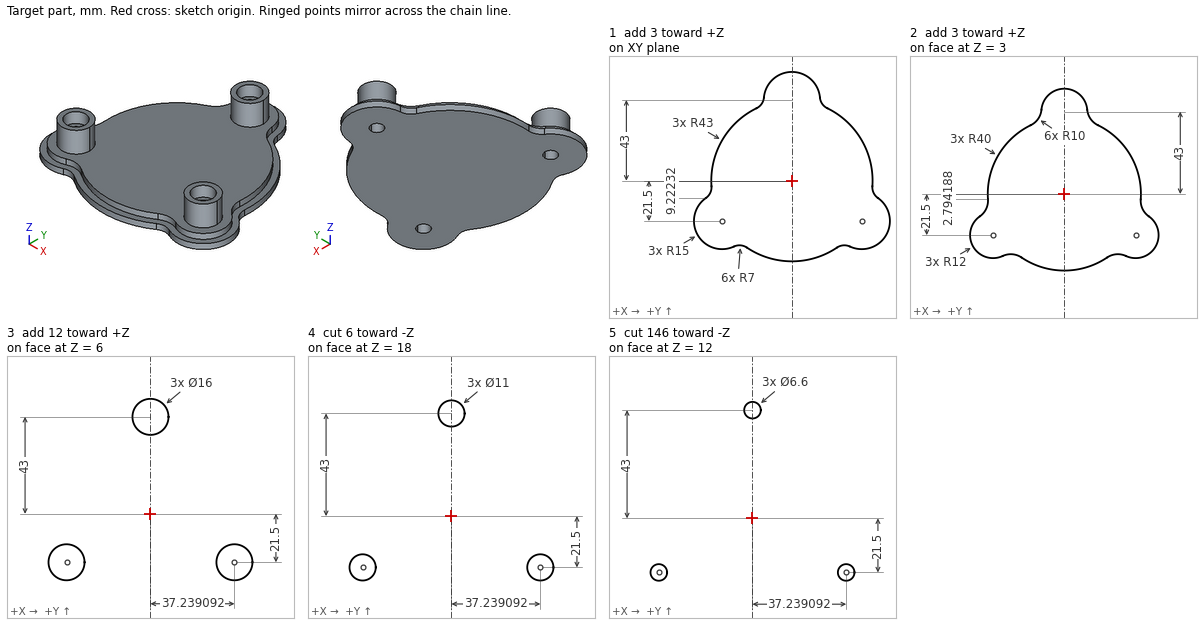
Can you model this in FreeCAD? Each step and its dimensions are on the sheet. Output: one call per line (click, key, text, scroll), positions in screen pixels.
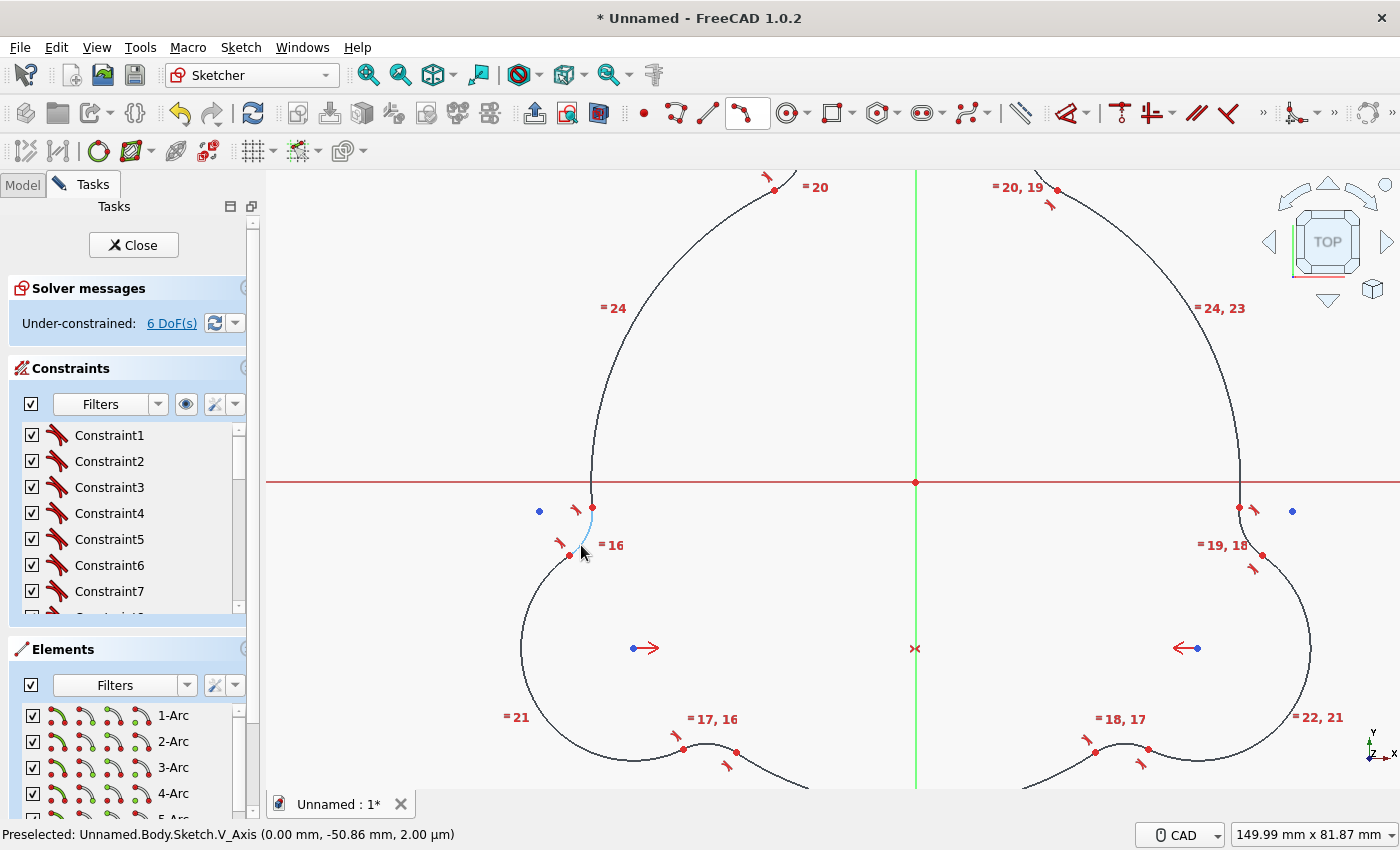
click(582, 544)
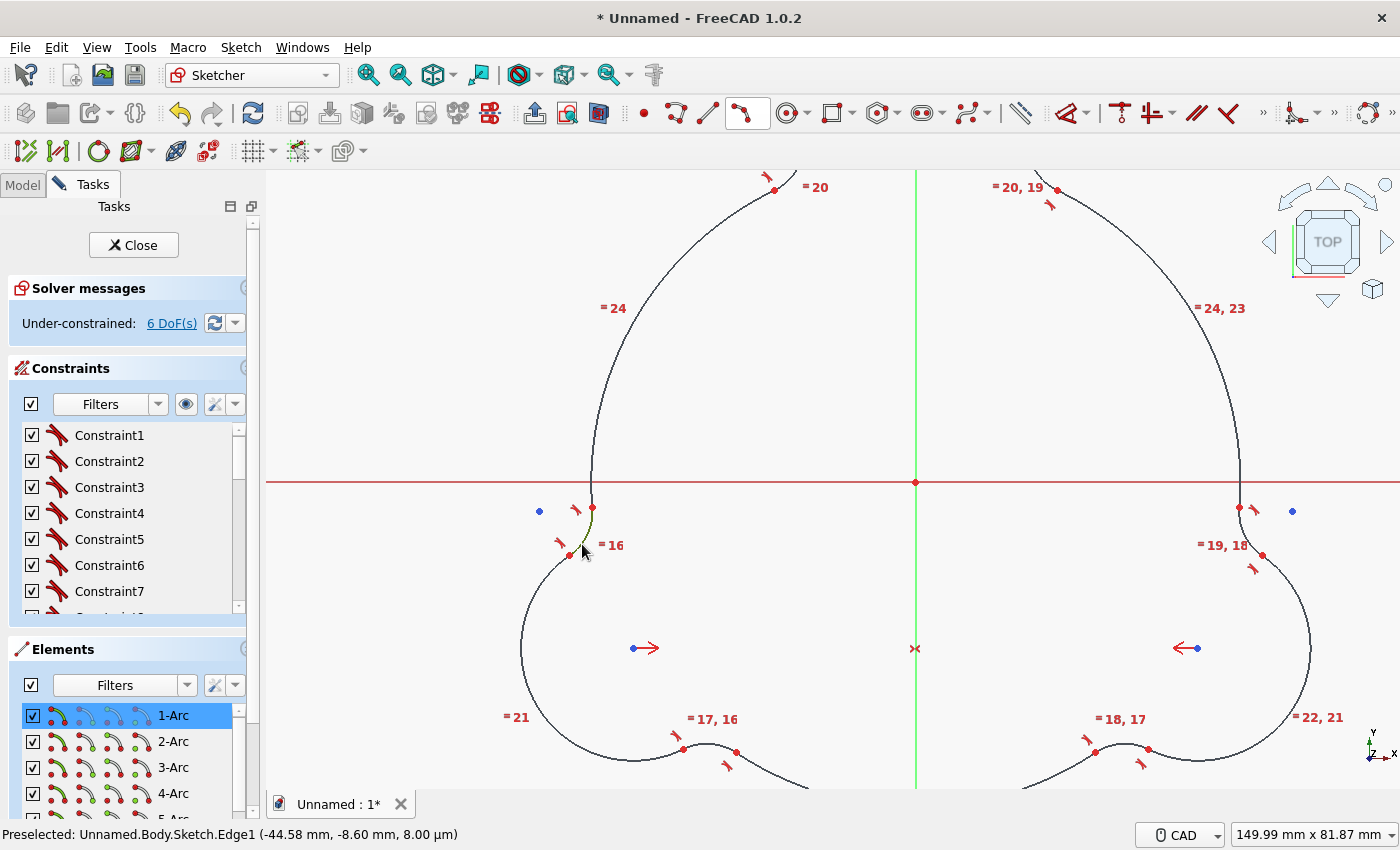
key(k)
key(r)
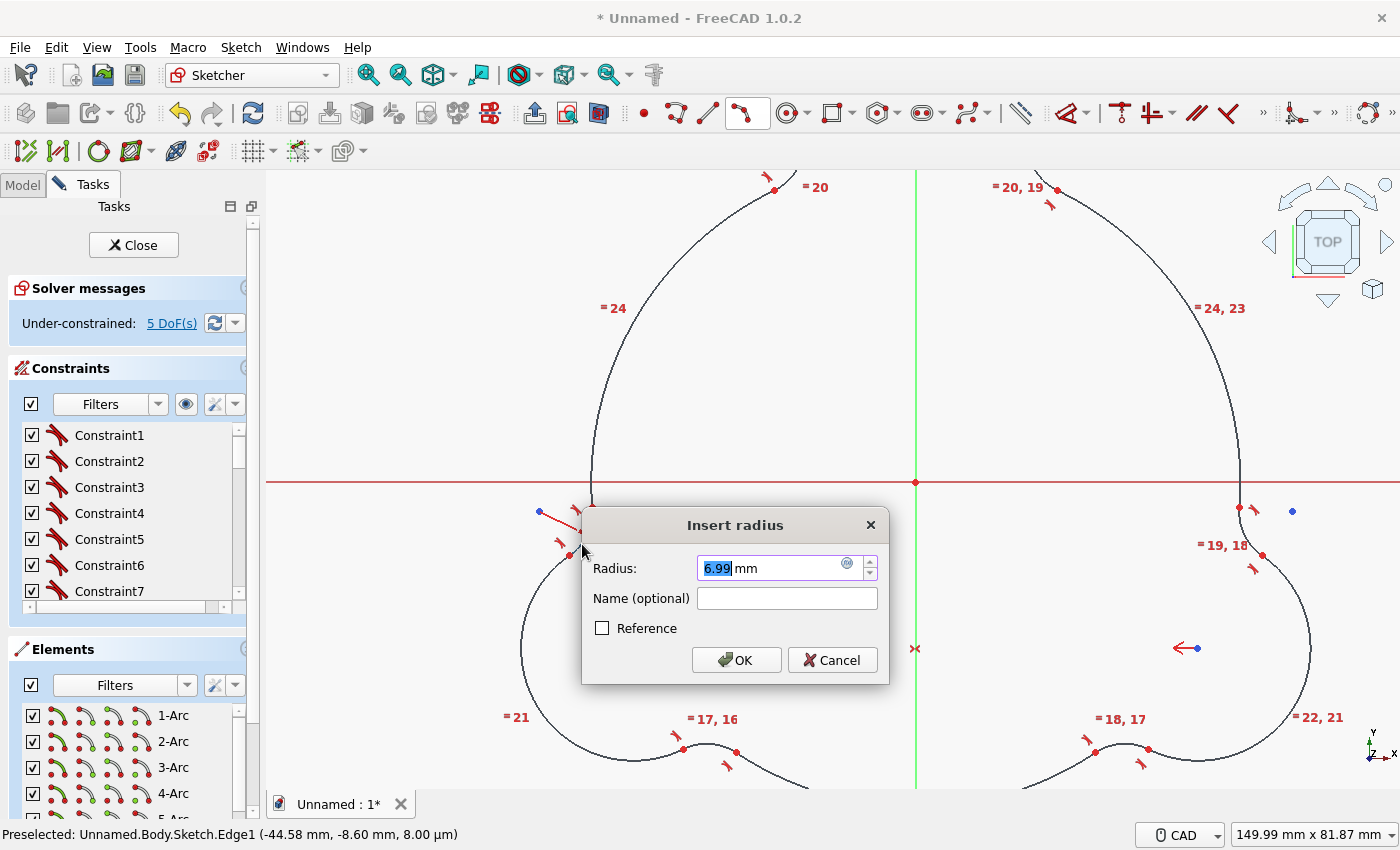
text(7)
key(Return)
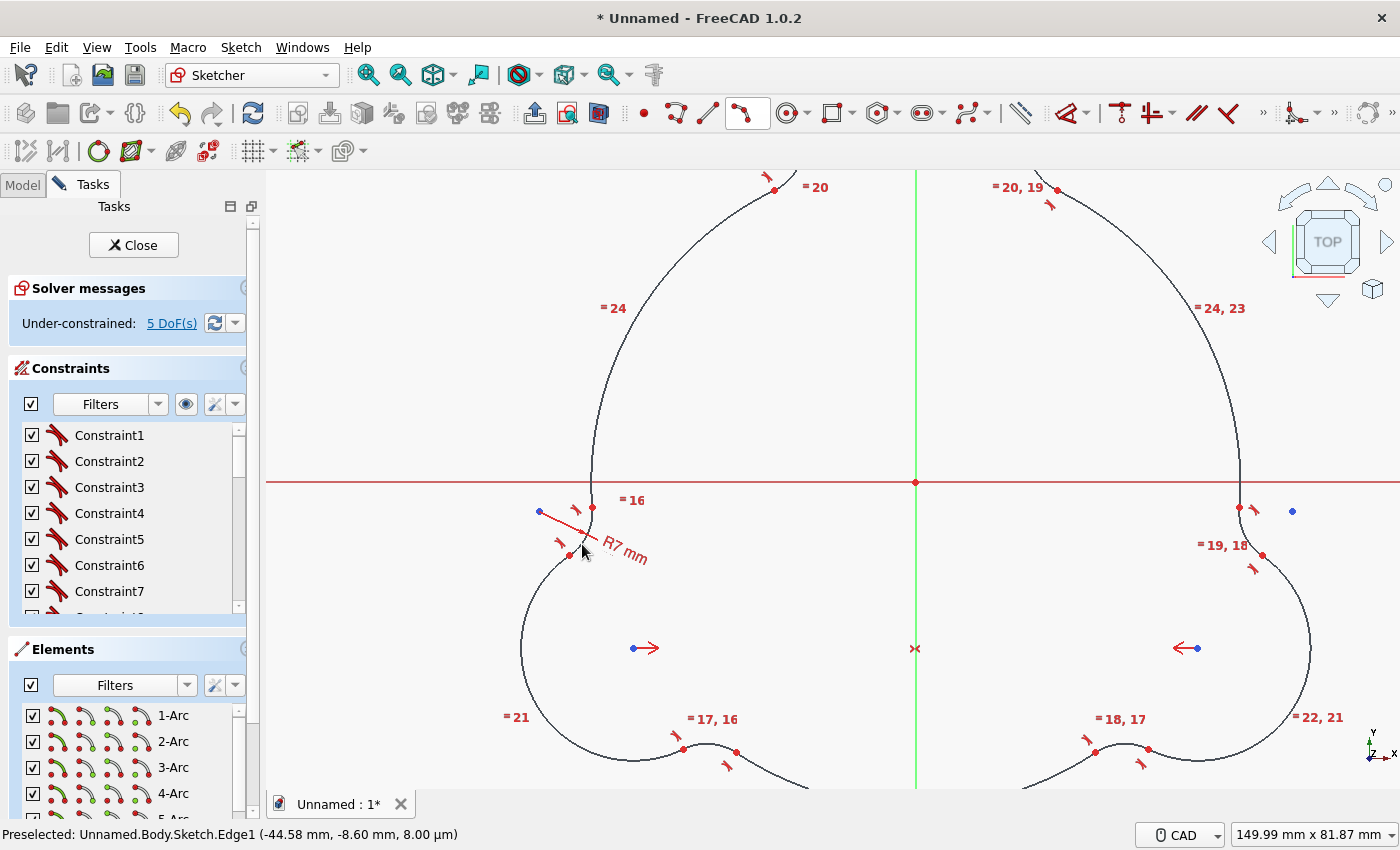
click(521, 640)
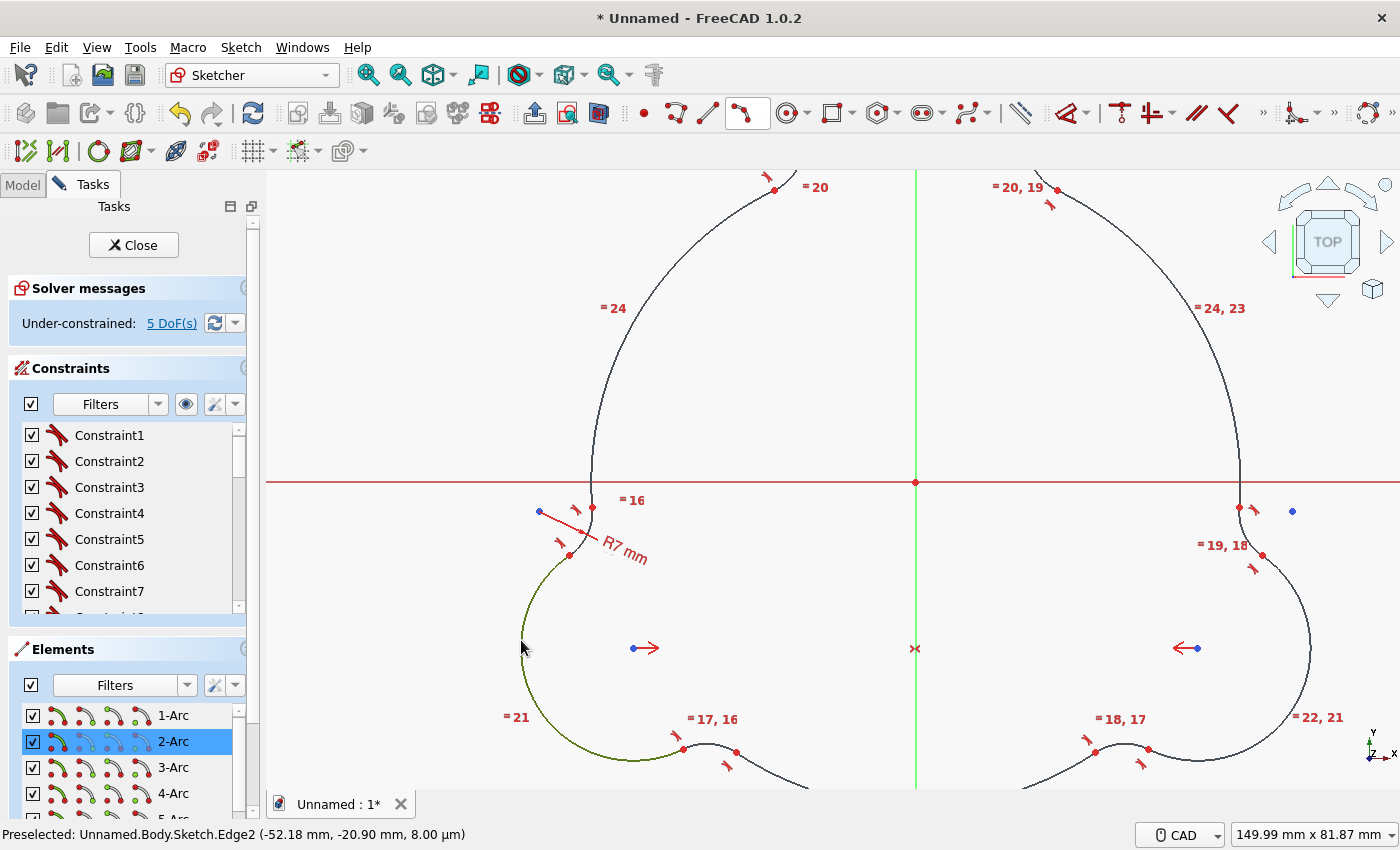
key(k)
key(r)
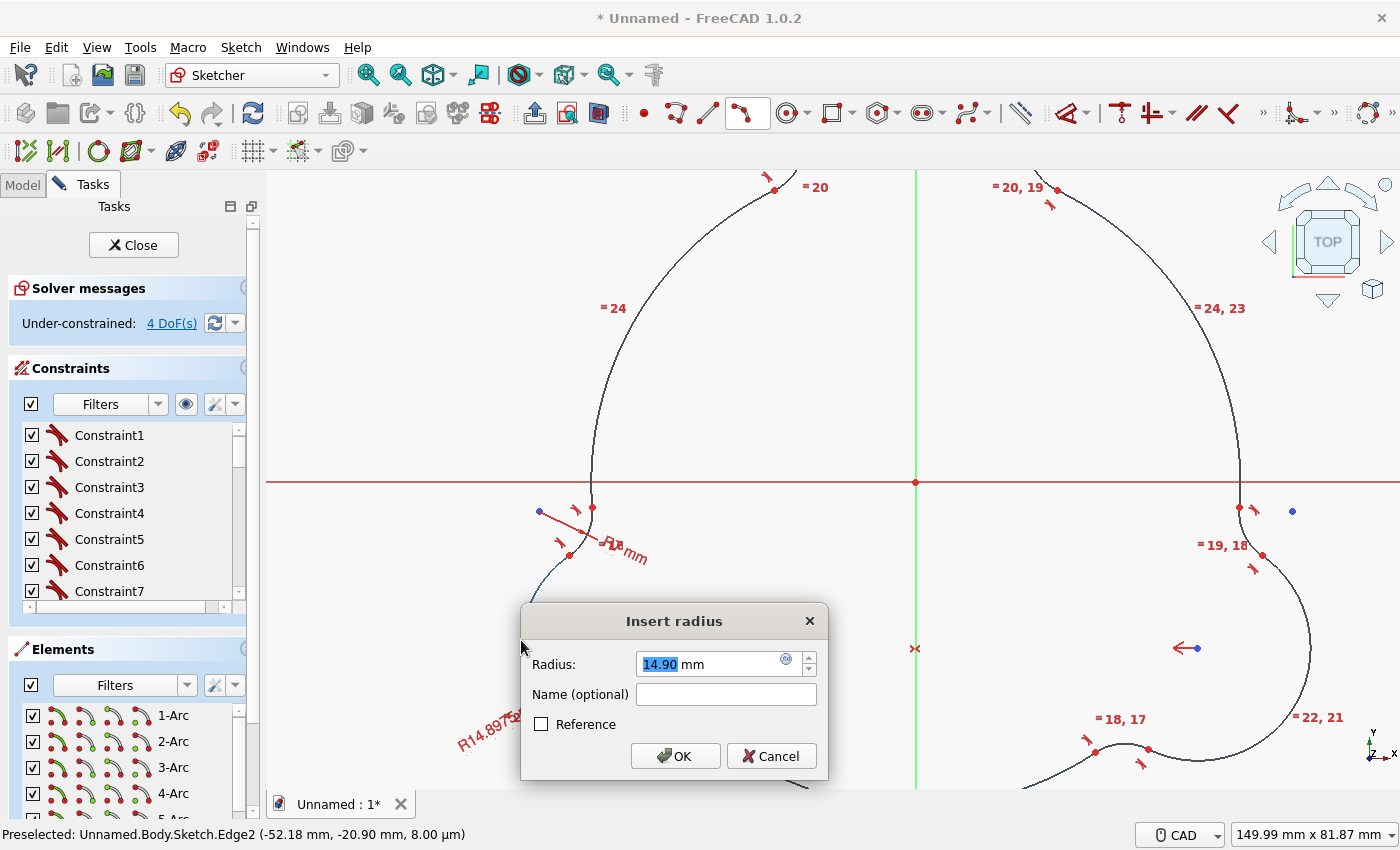
text(15)
key(Return)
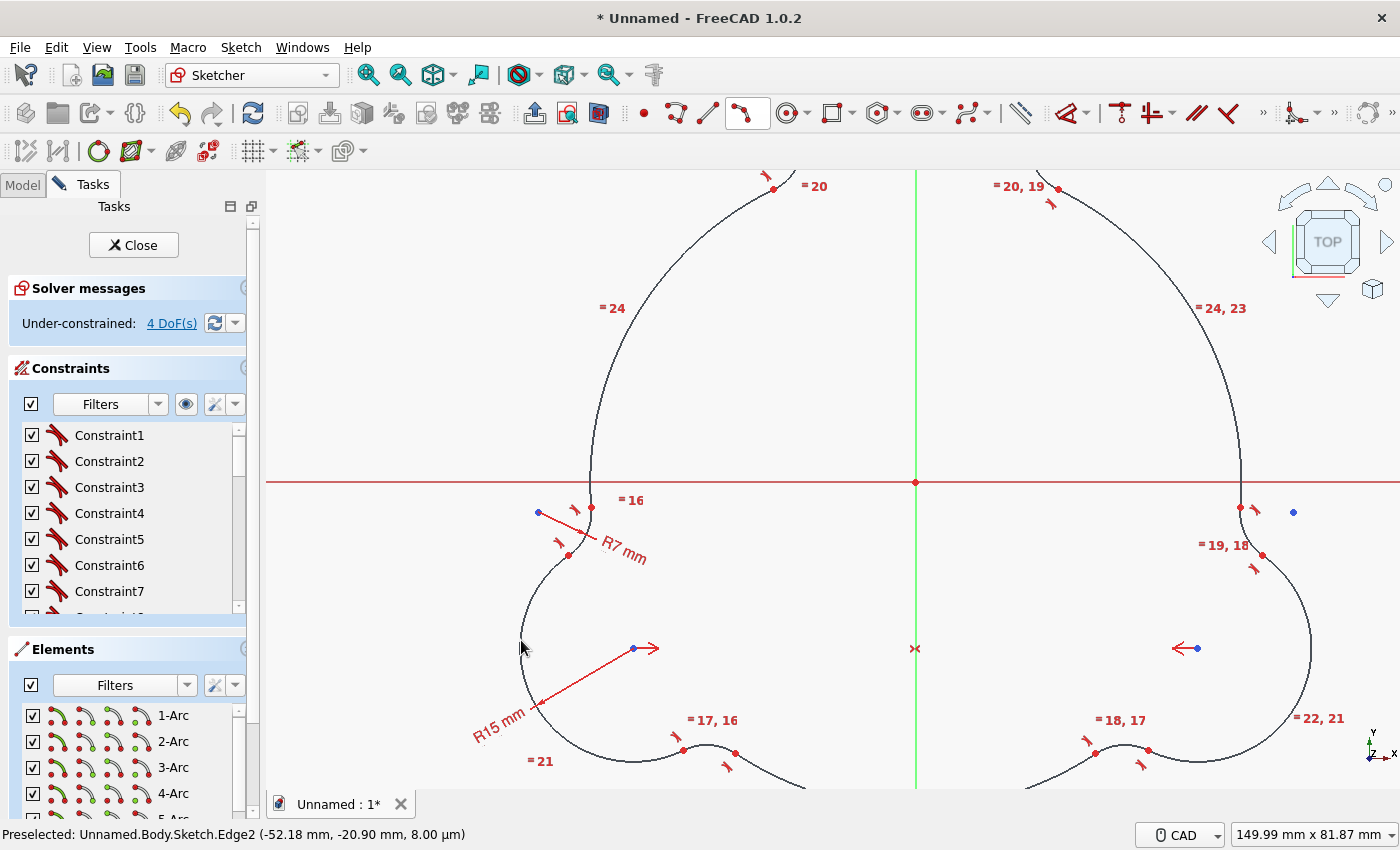
scroll(580, 545, down, 3)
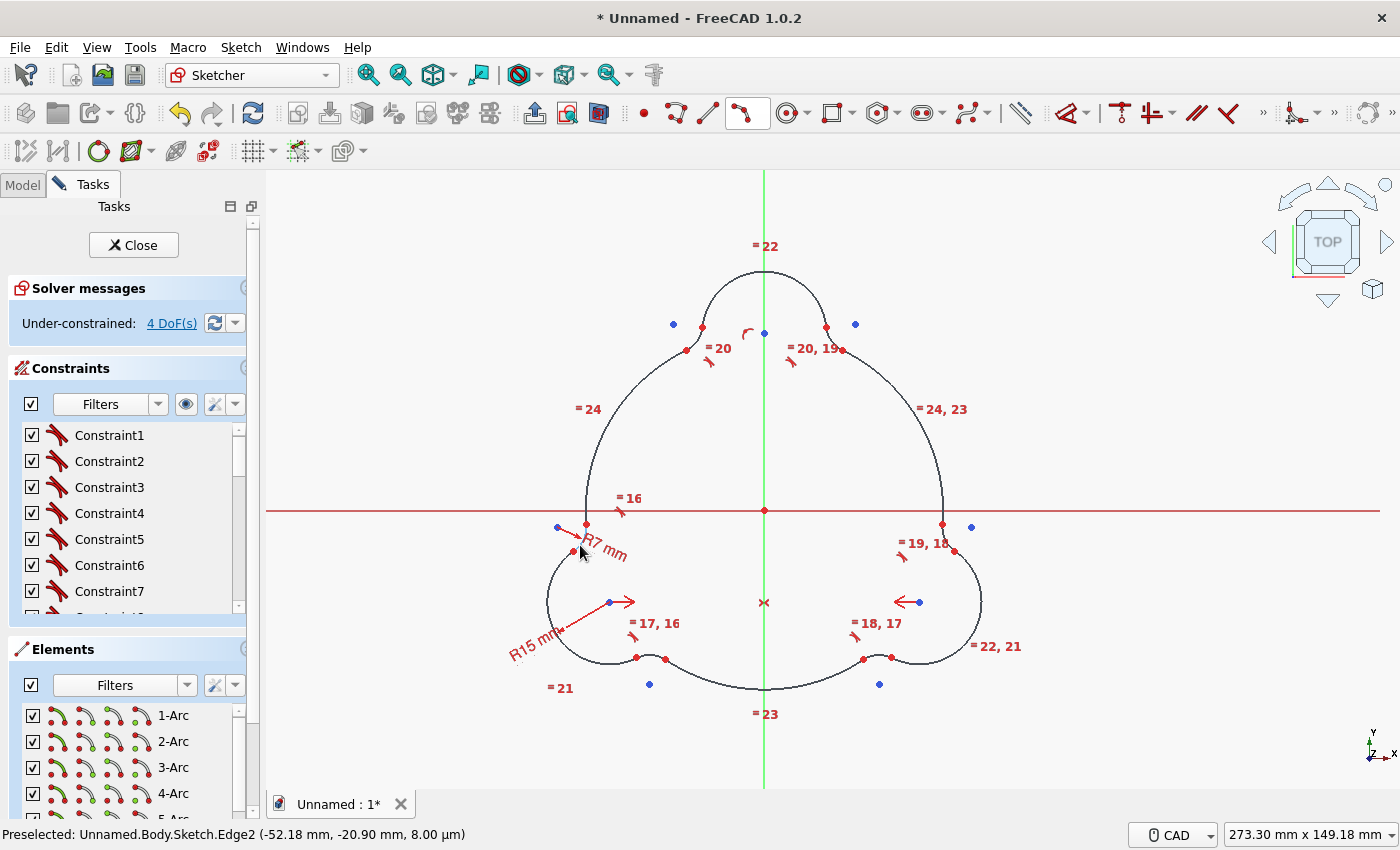
click(723, 685)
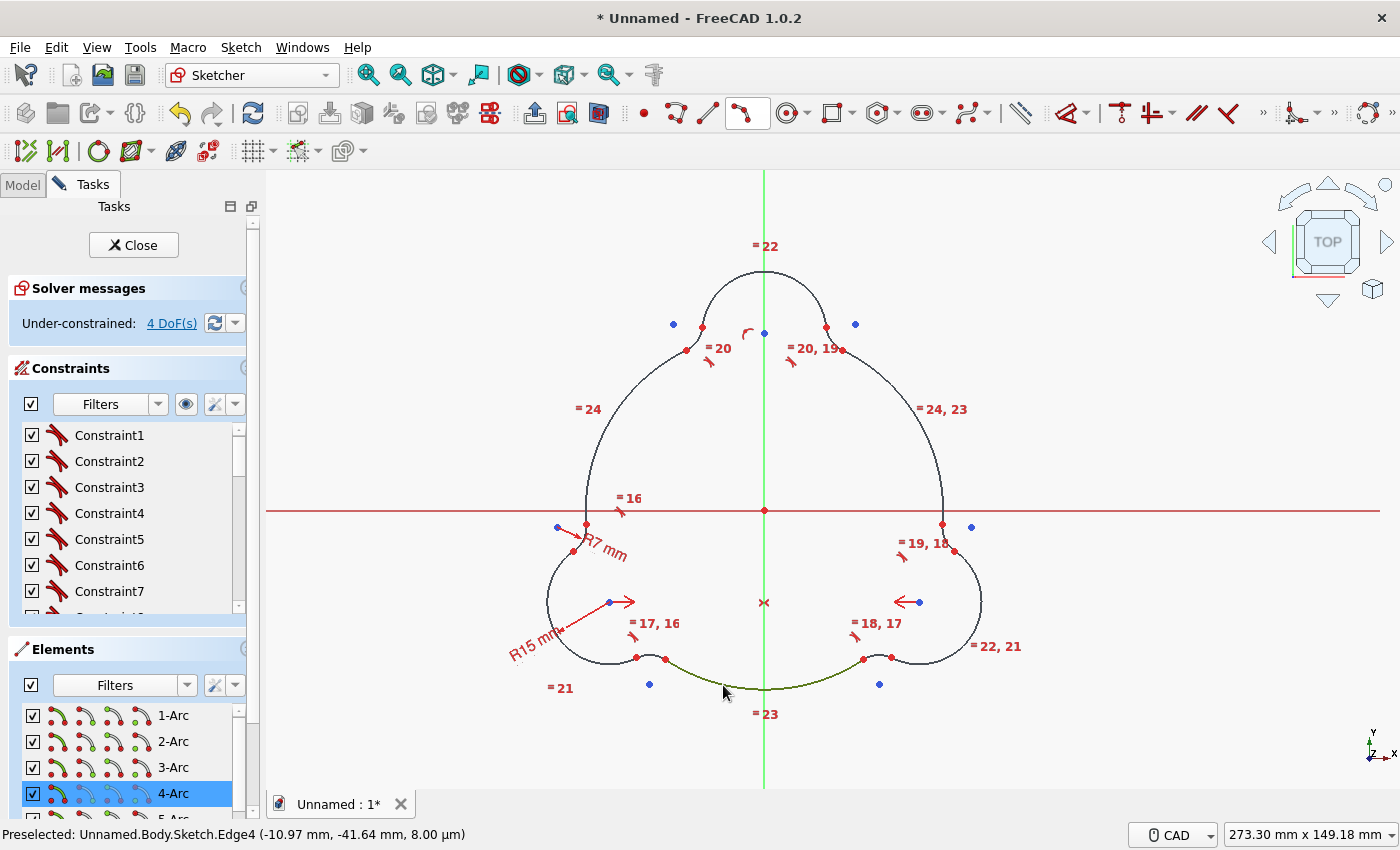
key(k)
key(r)